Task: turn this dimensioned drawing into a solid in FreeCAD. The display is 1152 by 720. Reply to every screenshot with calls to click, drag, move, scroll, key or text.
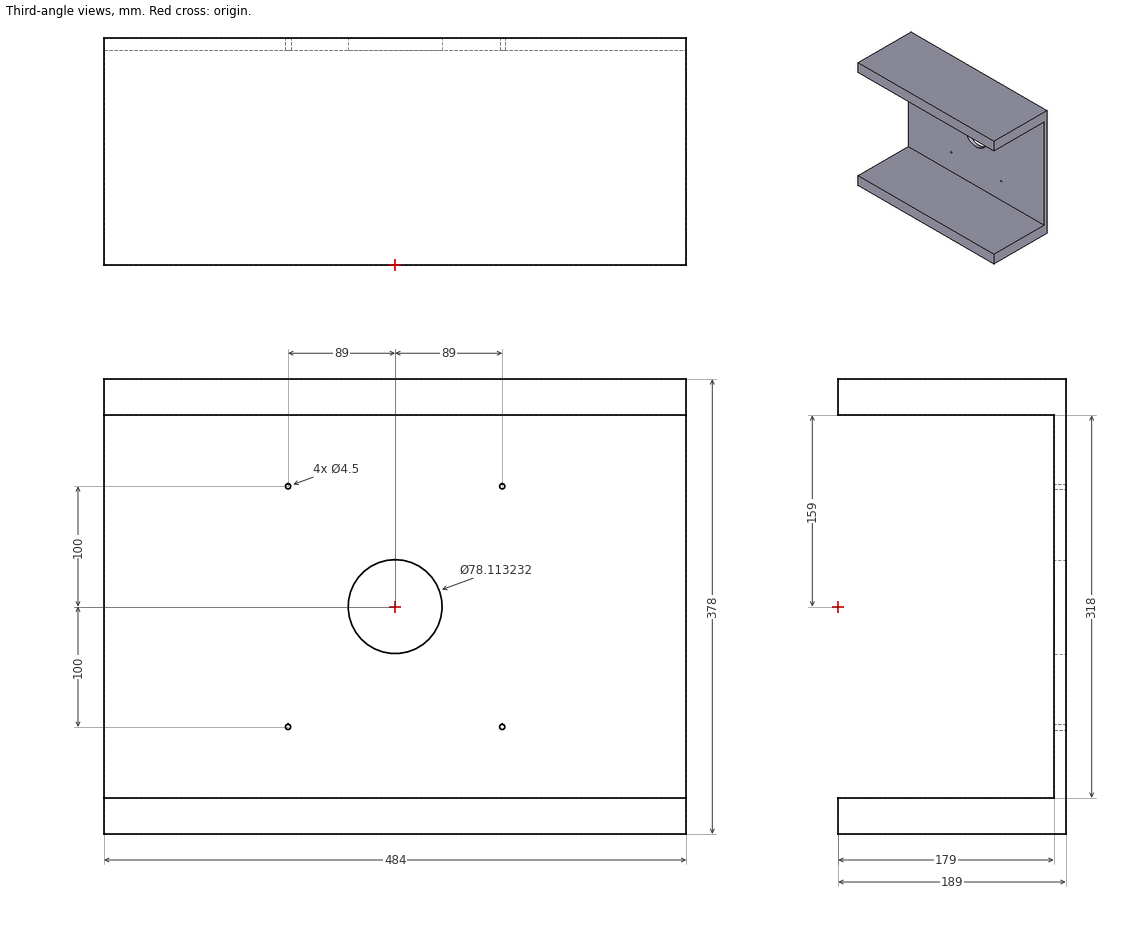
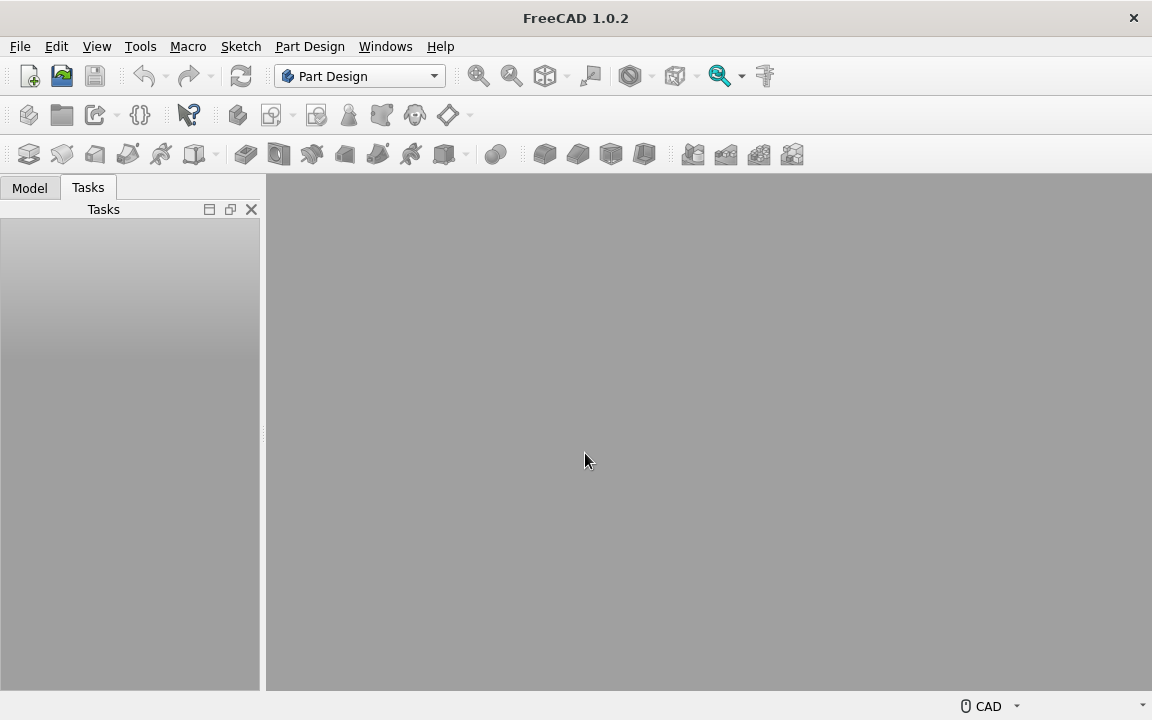
click(29, 76)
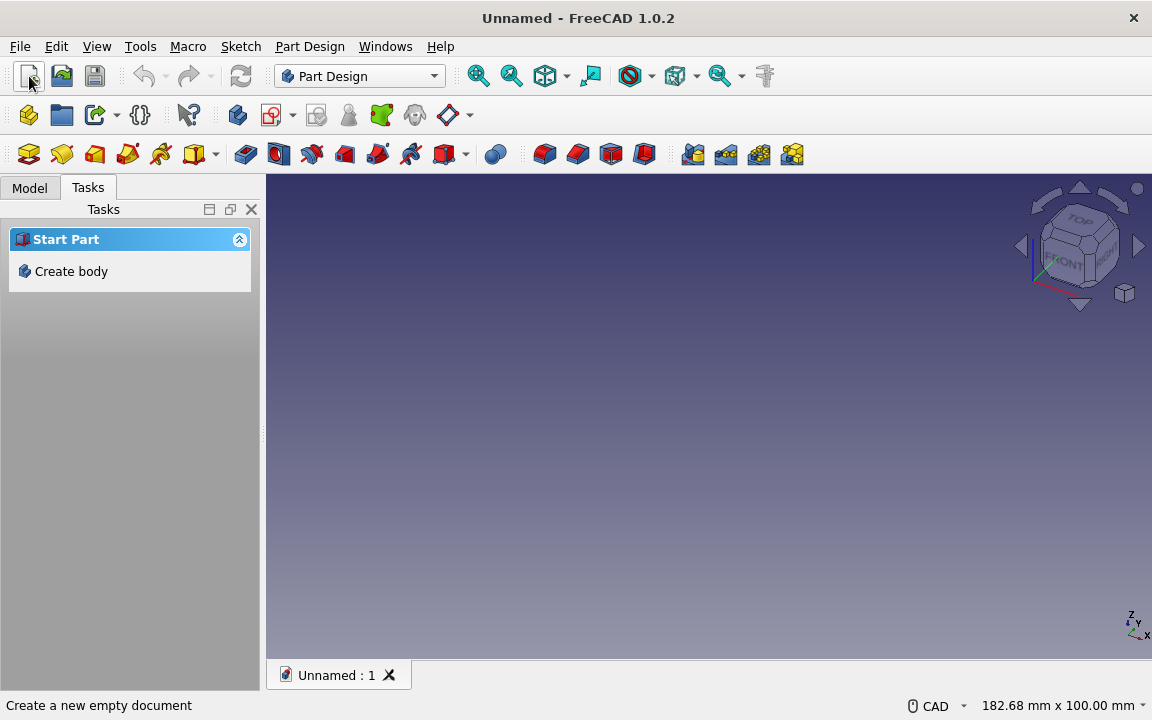
click(270, 116)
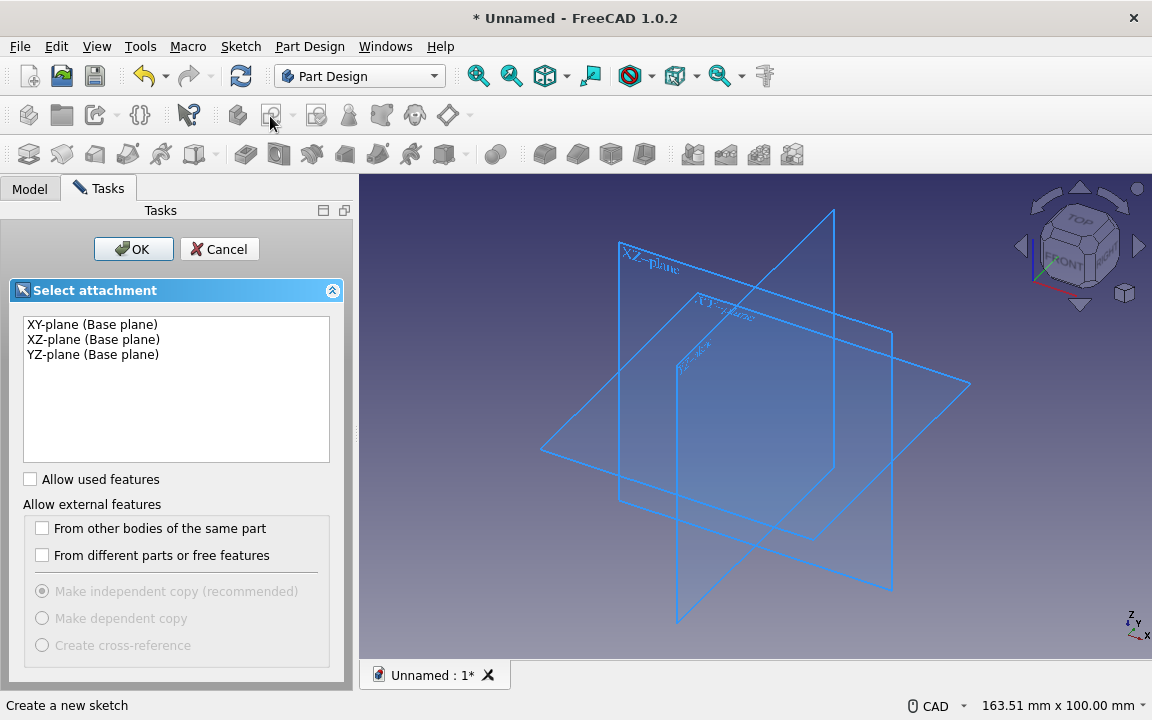
click(84, 340)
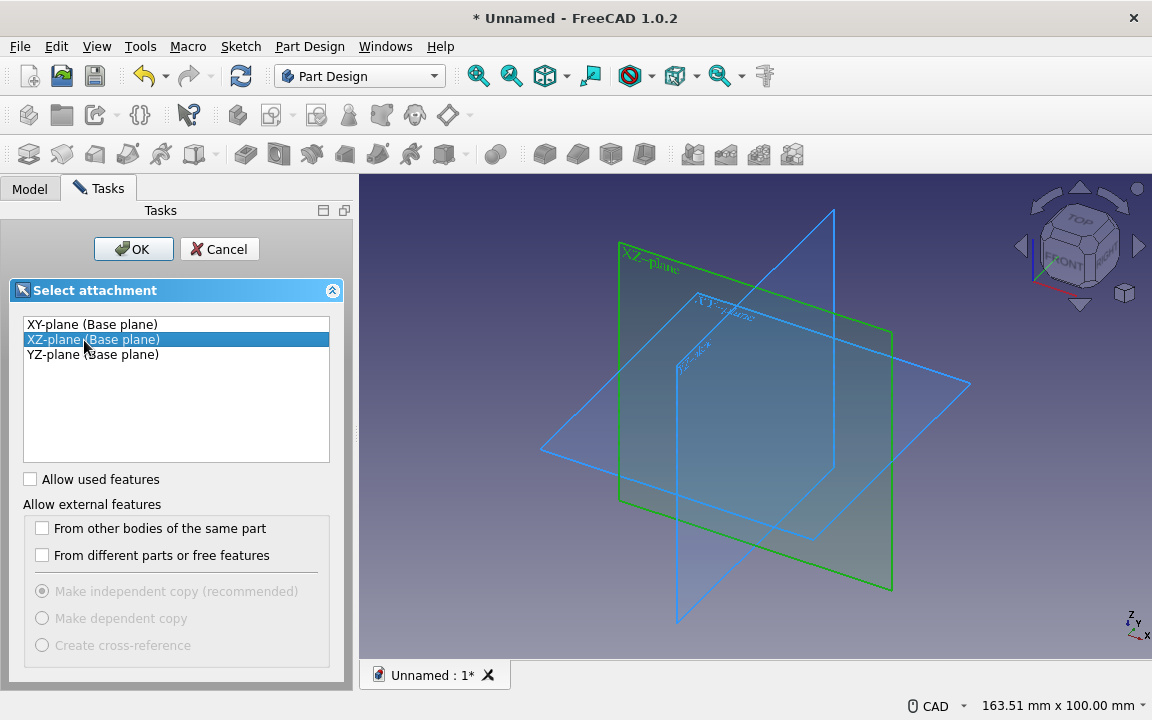
click(134, 249)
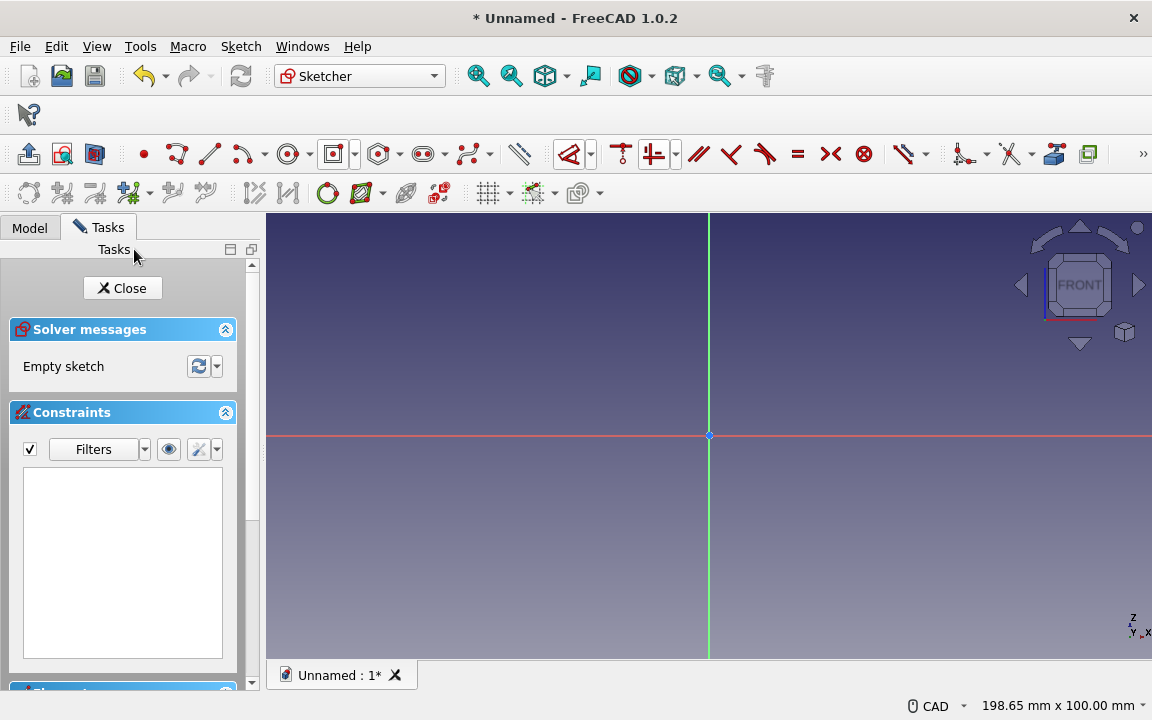
scroll(627, 436, down, 9)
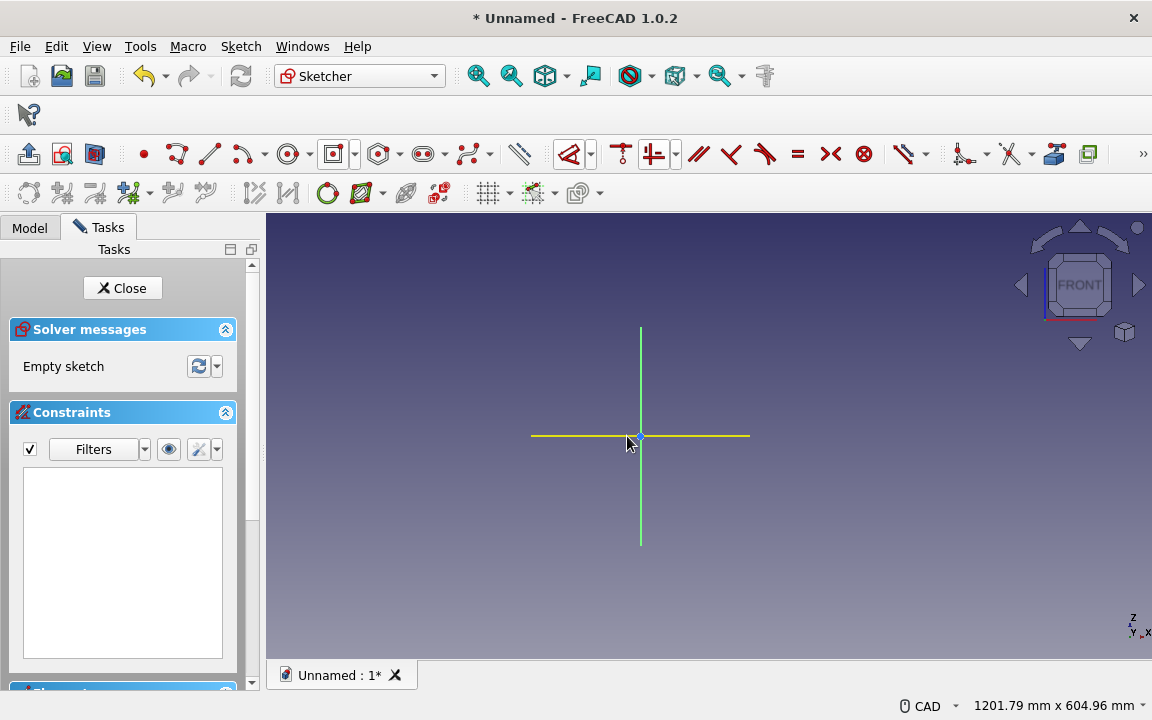
click(332, 154)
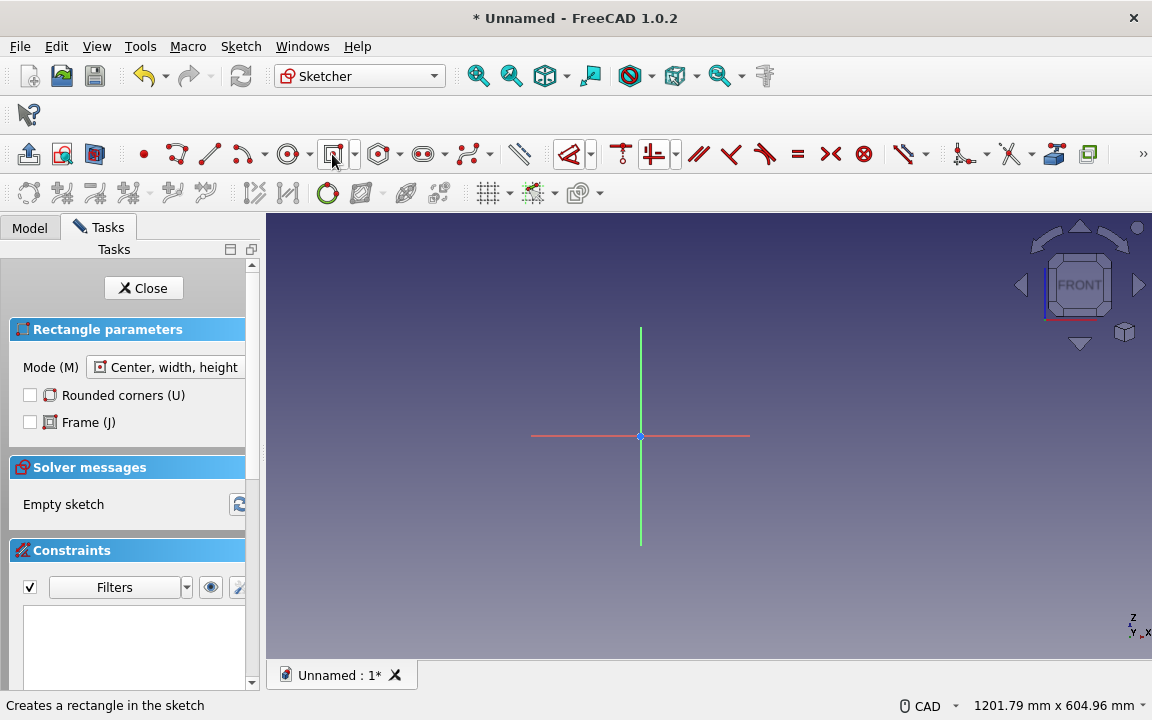
click(641, 436)
move(819, 297)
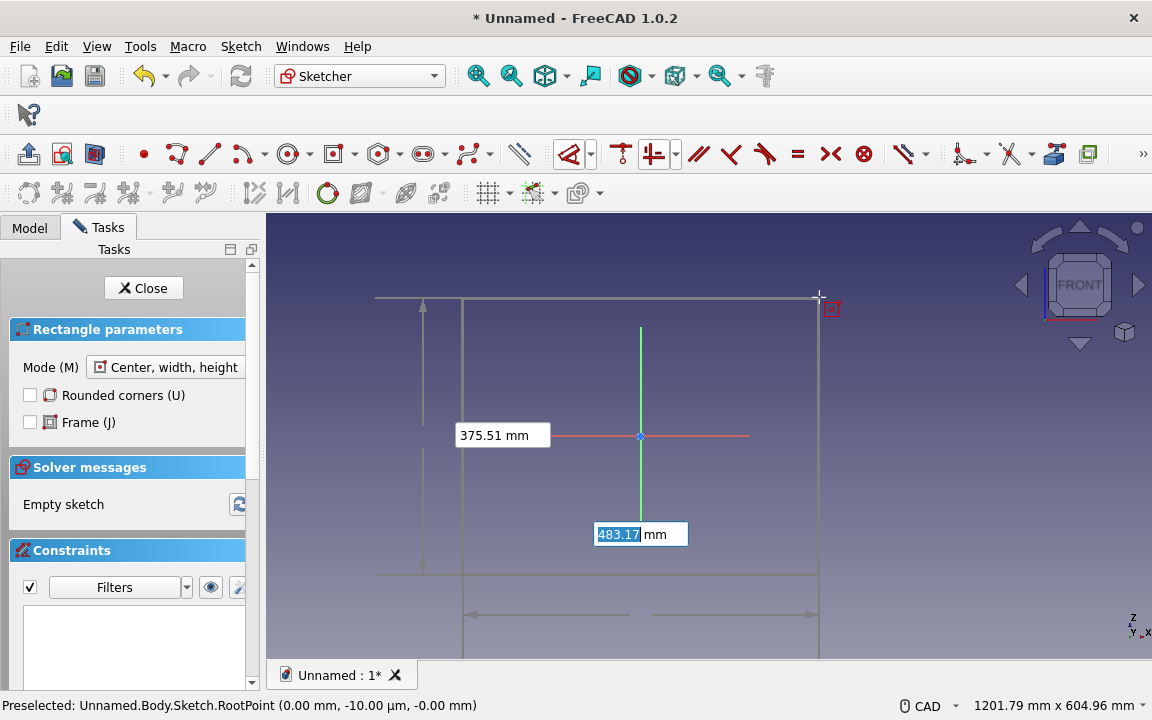
text(484)
key(Tab)
text(378)
key(Return)
key(Escape)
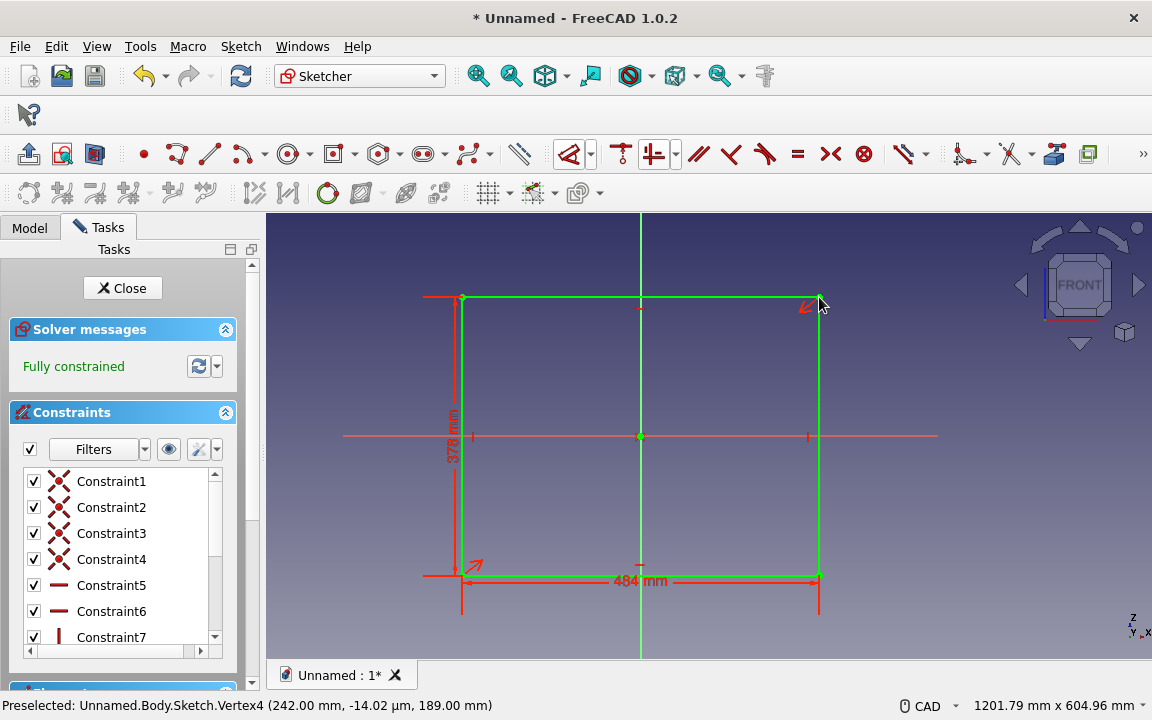
click(123, 288)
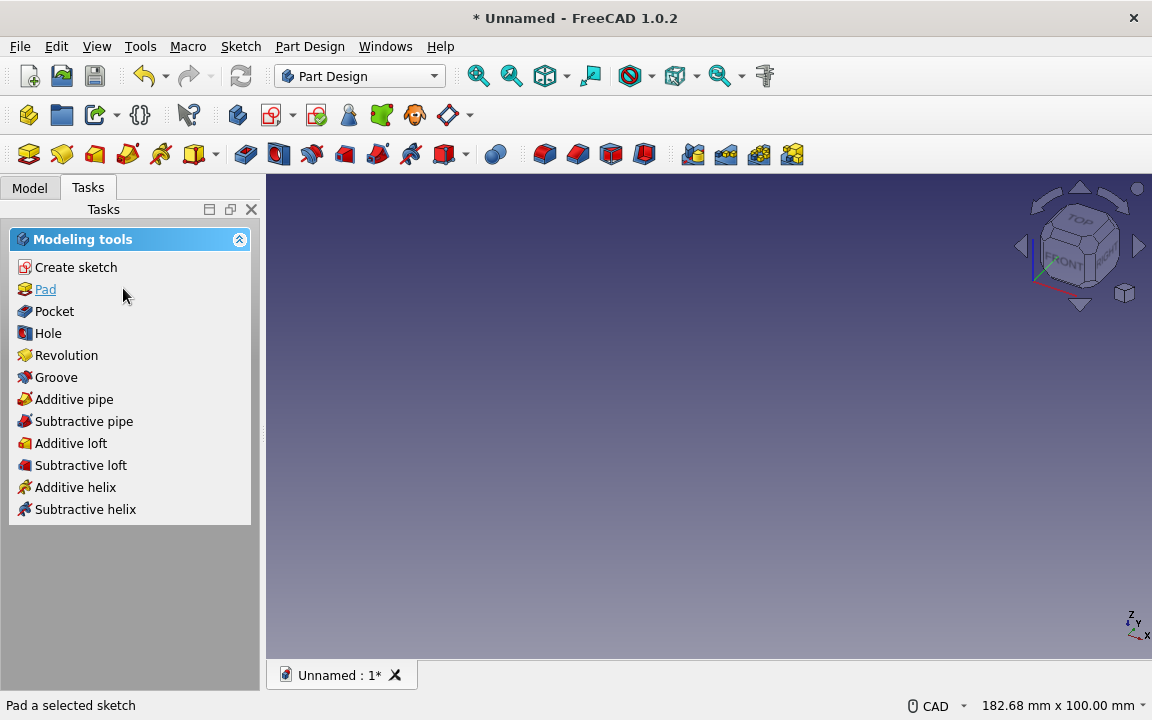
click(29, 154)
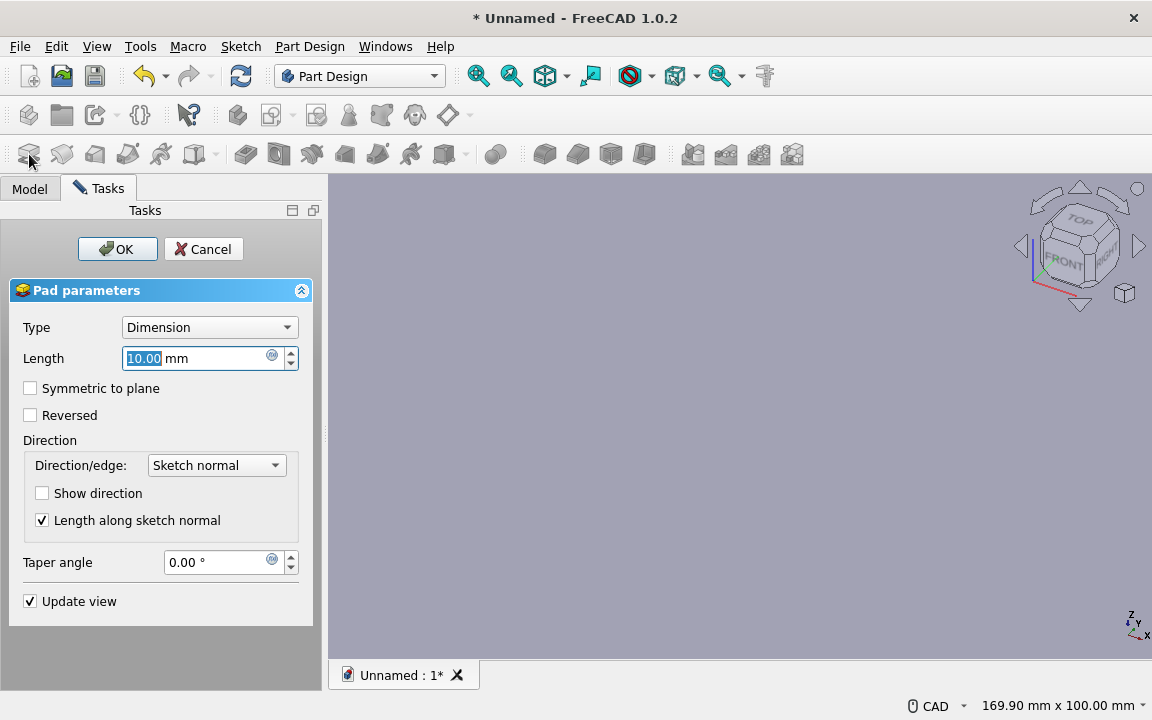
text(189)
key(Tab)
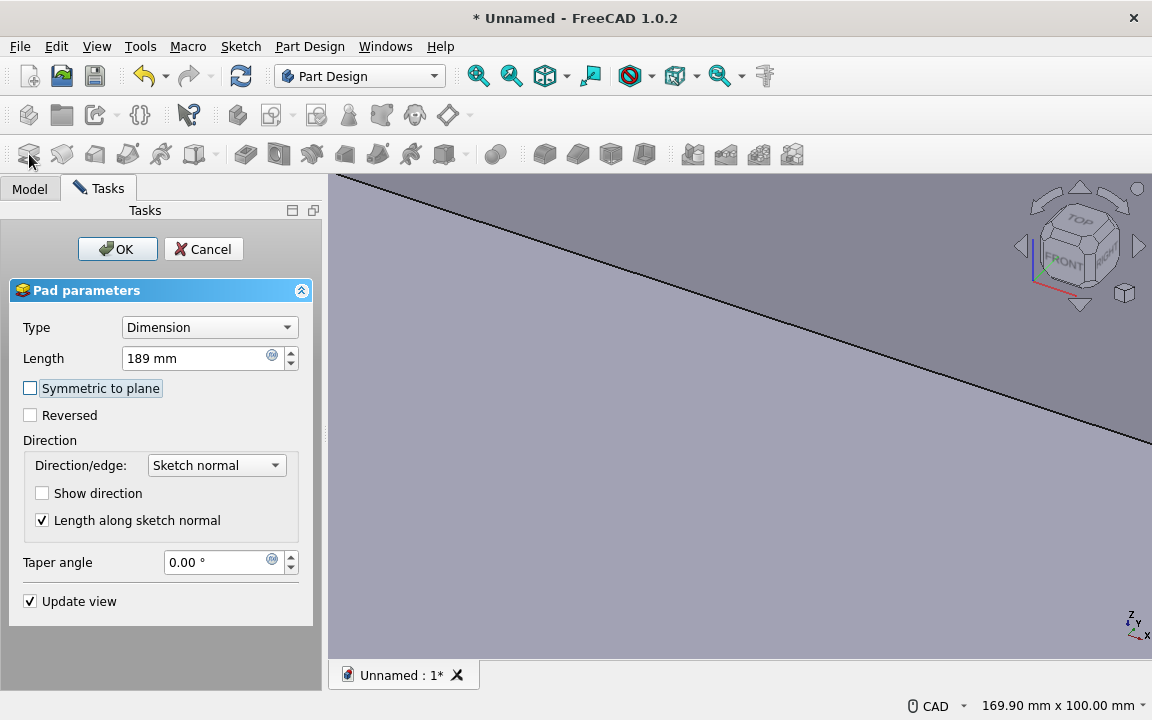
click(31, 415)